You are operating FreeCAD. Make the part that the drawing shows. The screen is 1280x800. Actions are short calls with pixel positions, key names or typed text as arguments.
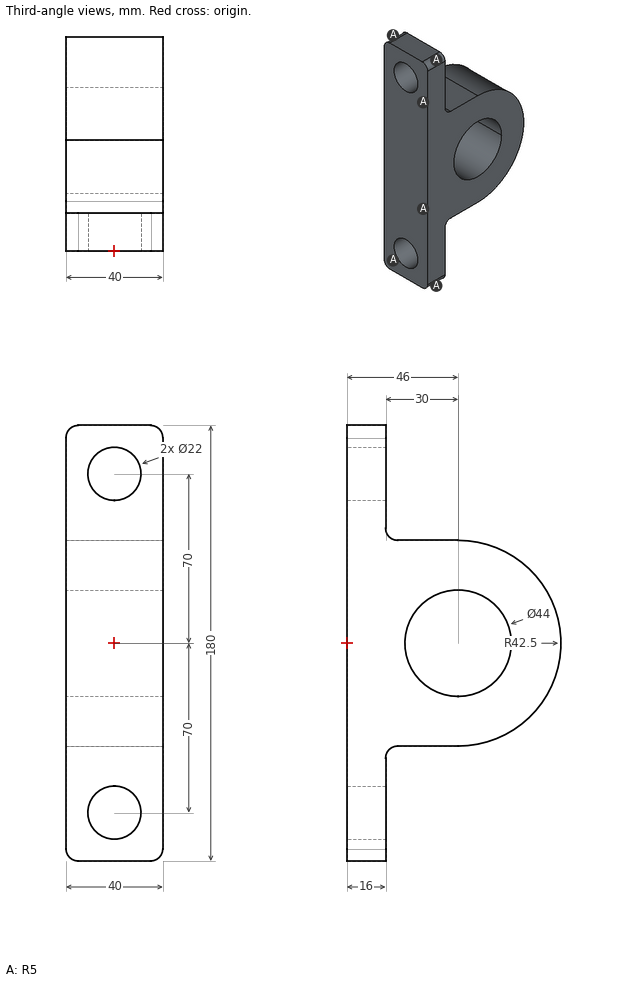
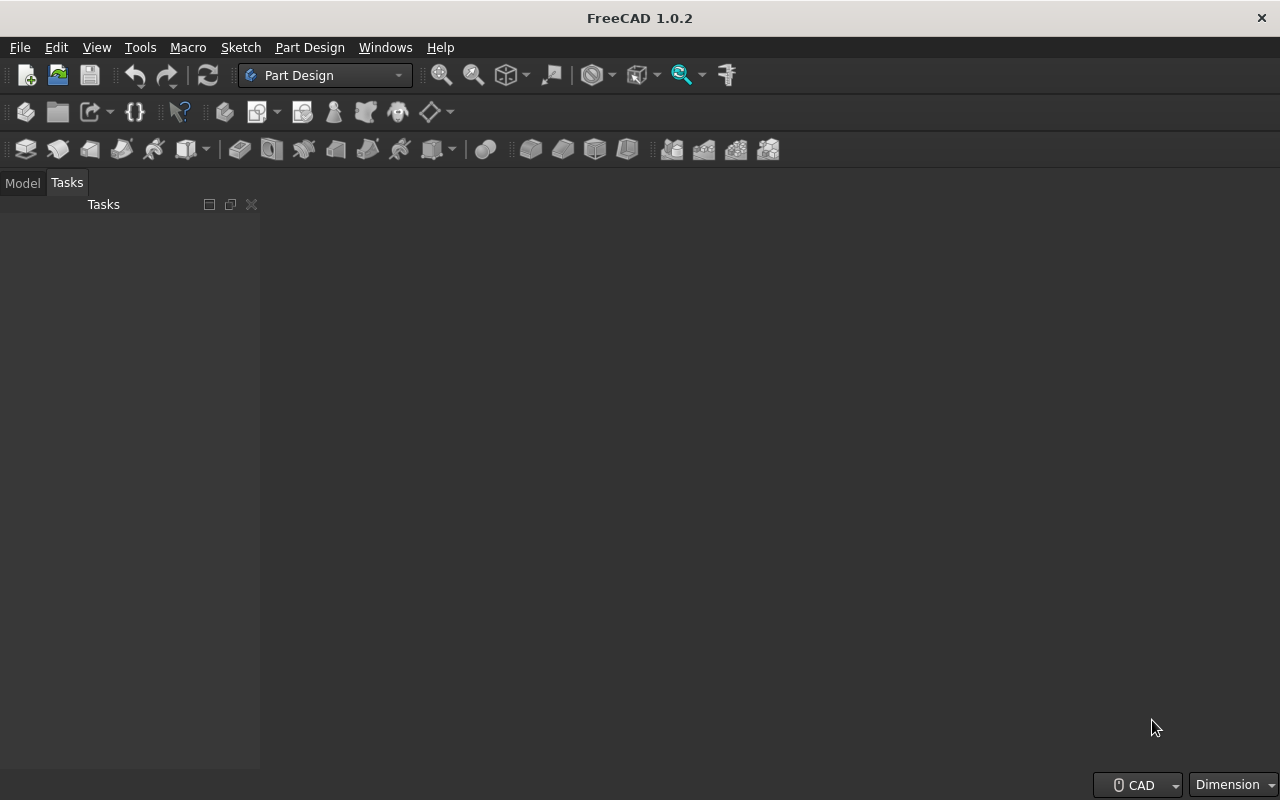
click(26, 76)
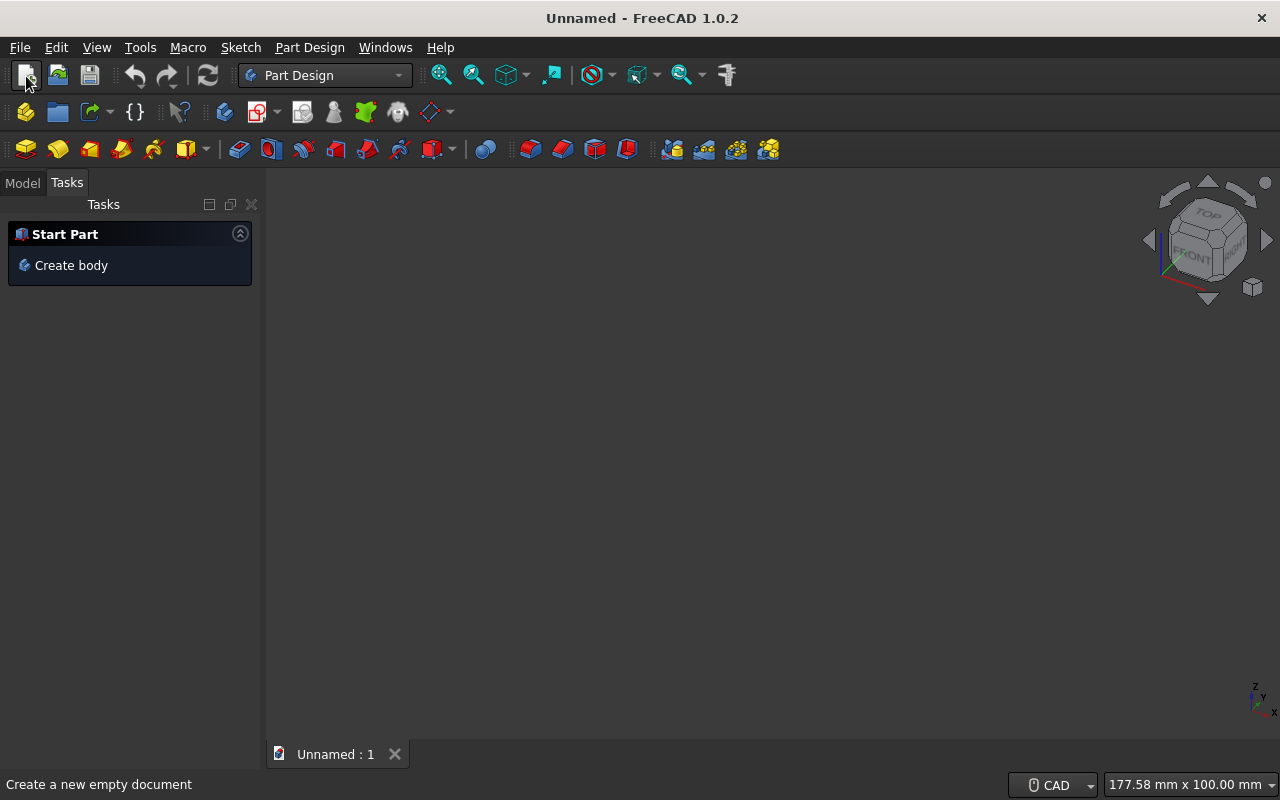
click(258, 112)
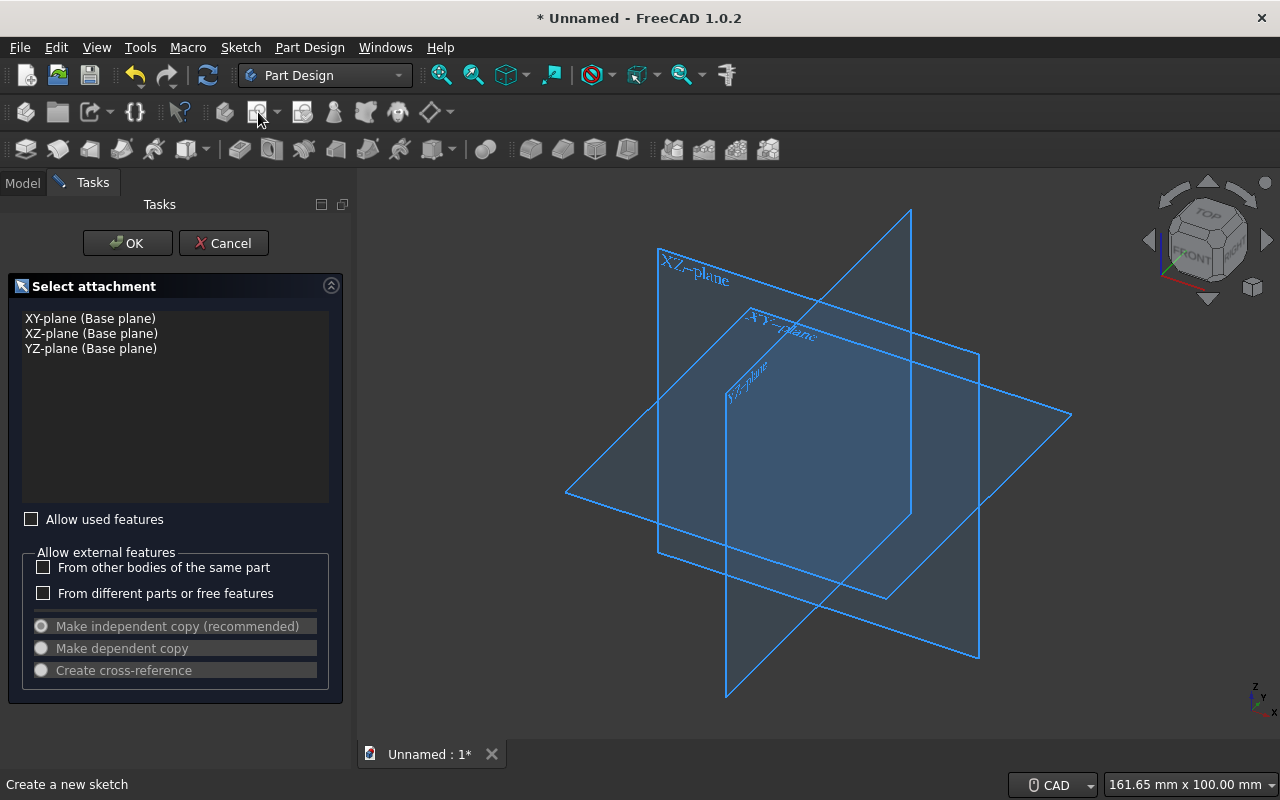
click(82, 334)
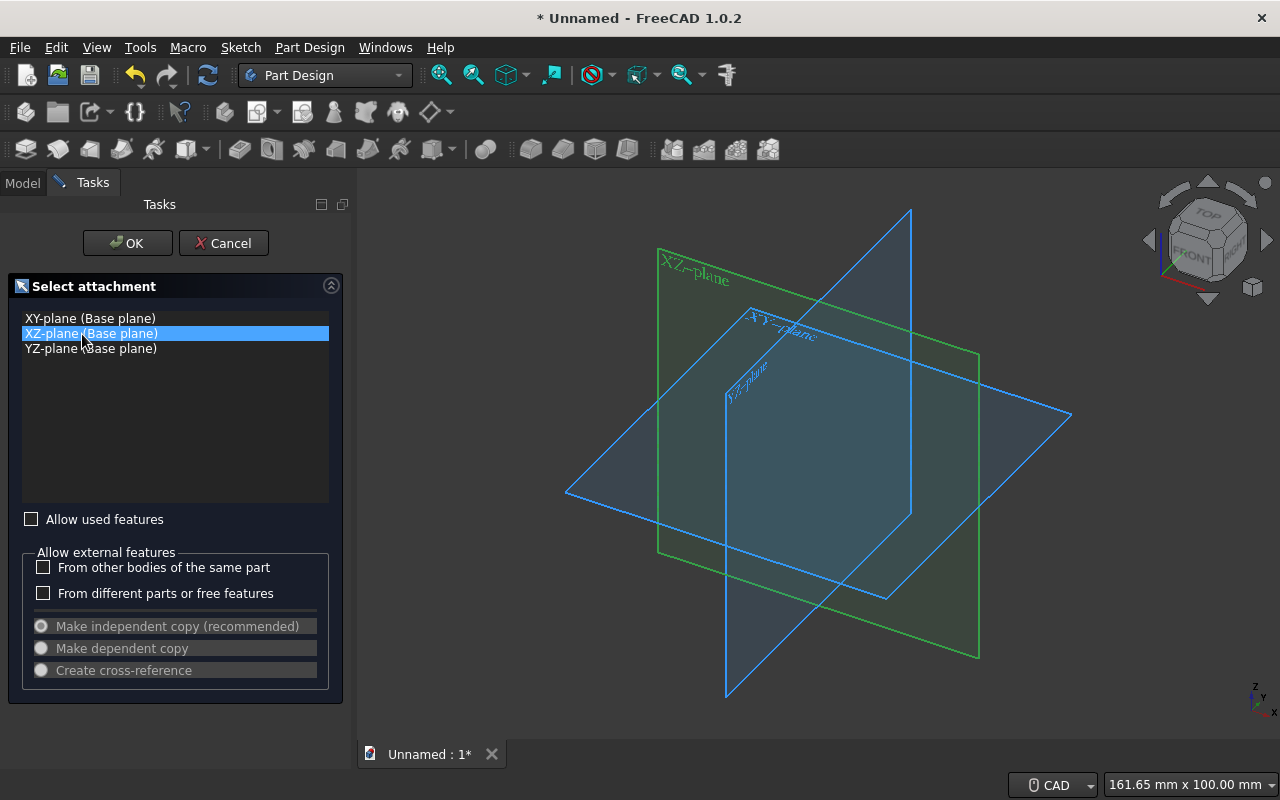
click(128, 243)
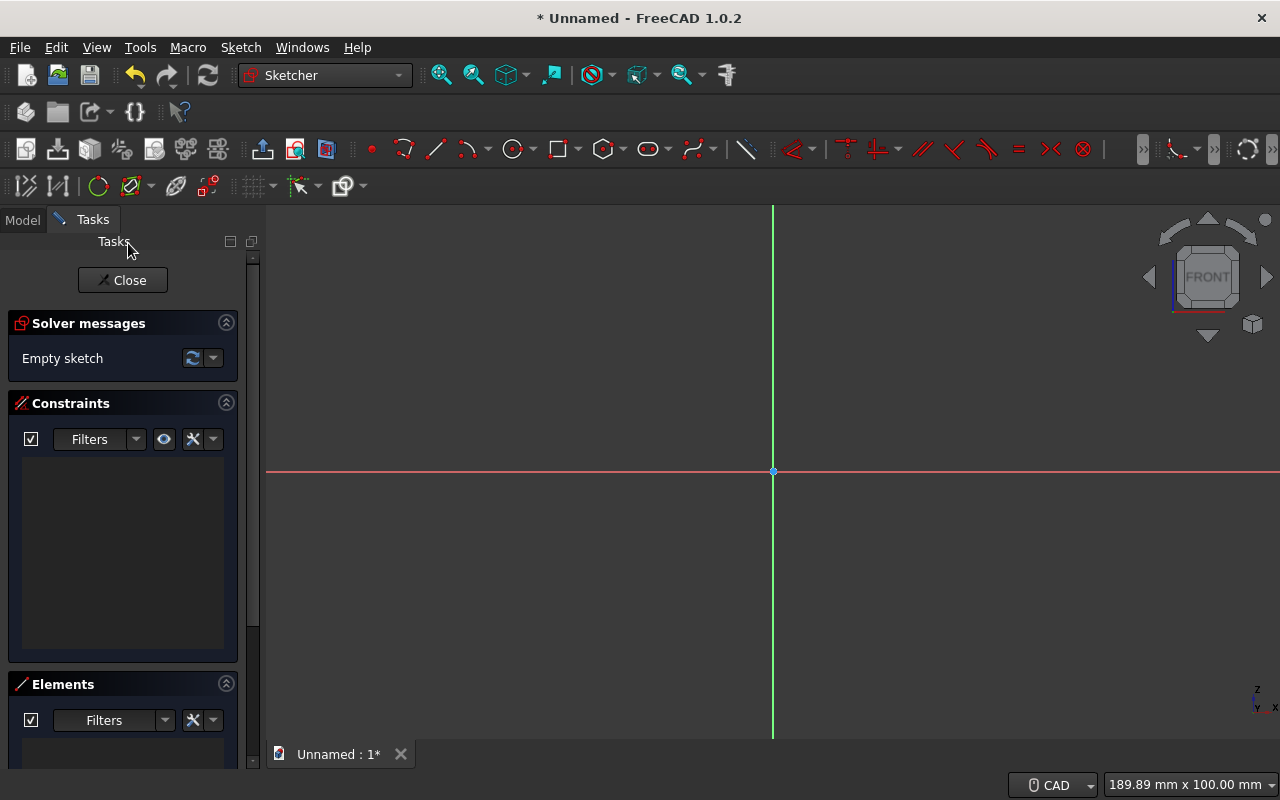
scroll(665, 472, down, 5)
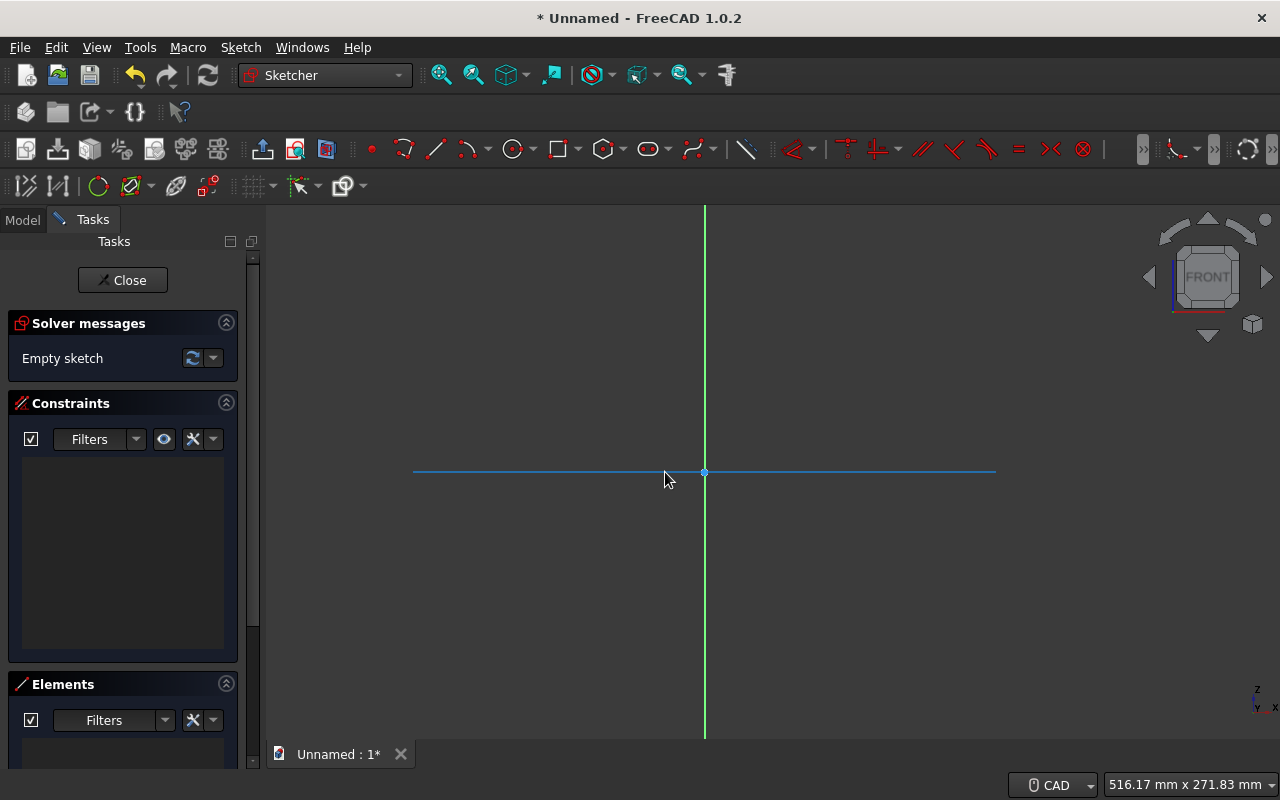
key(g)
key(v)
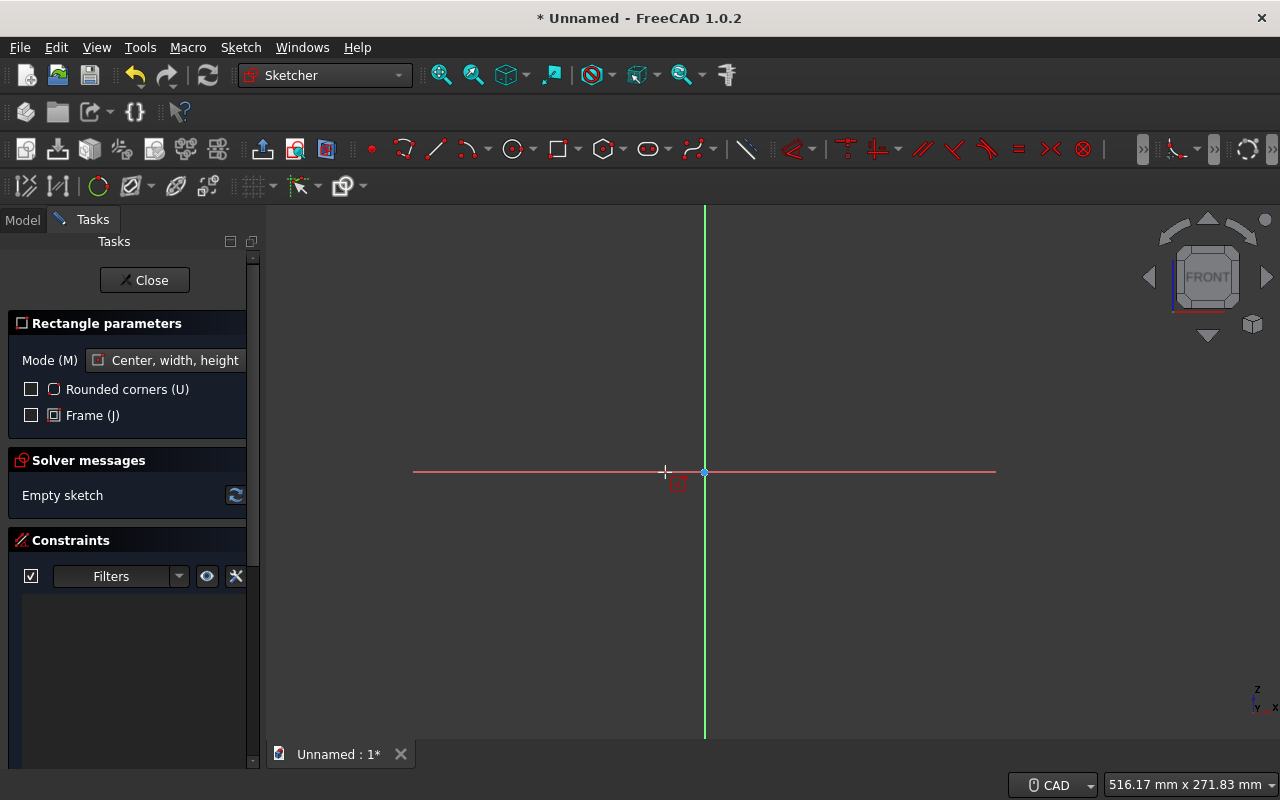
click(705, 472)
click(744, 296)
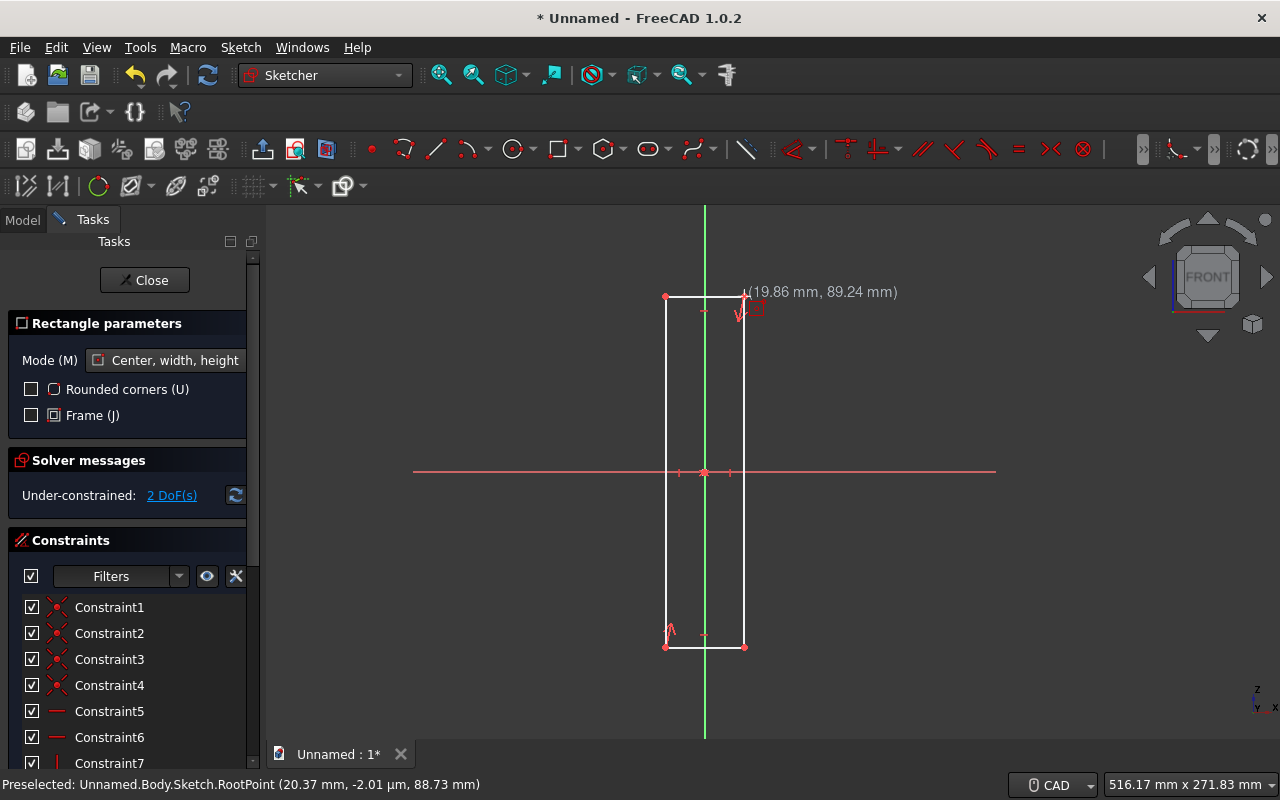
key(g)
key(c)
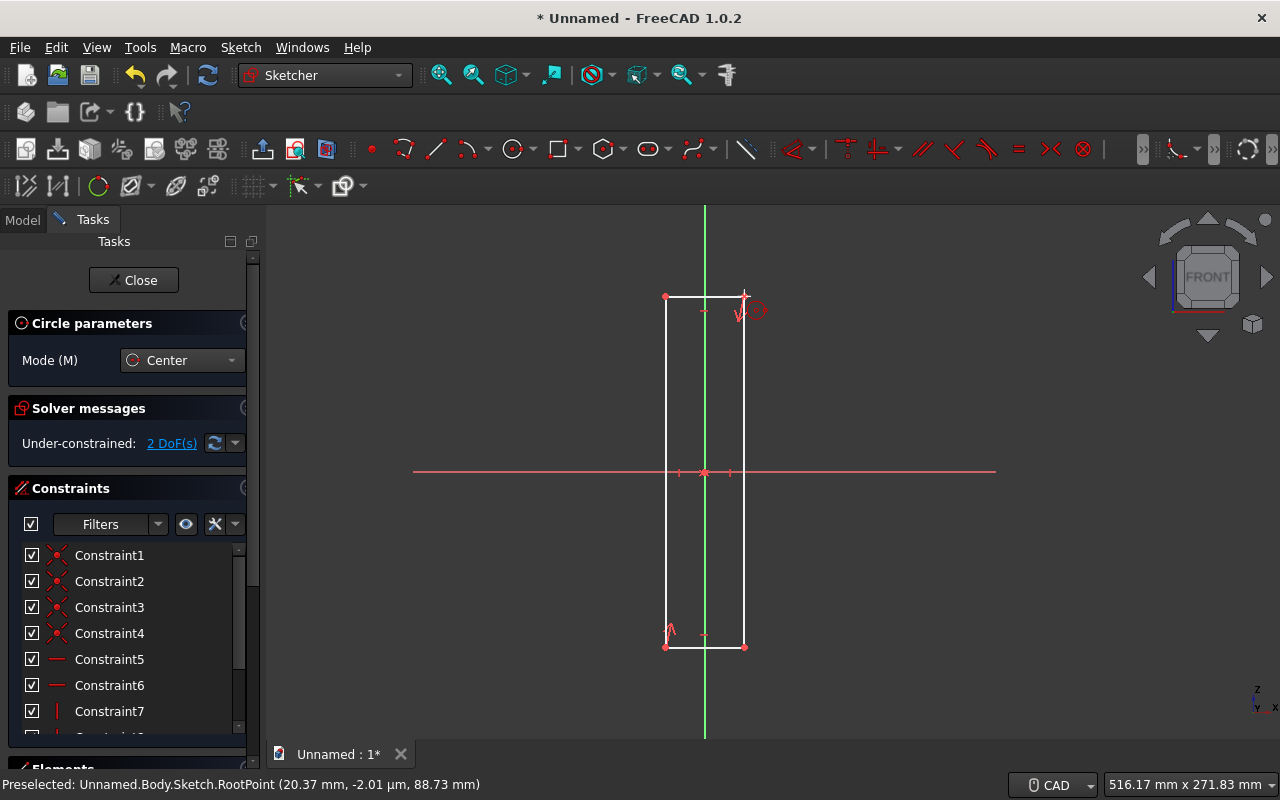
click(705, 335)
click(720, 320)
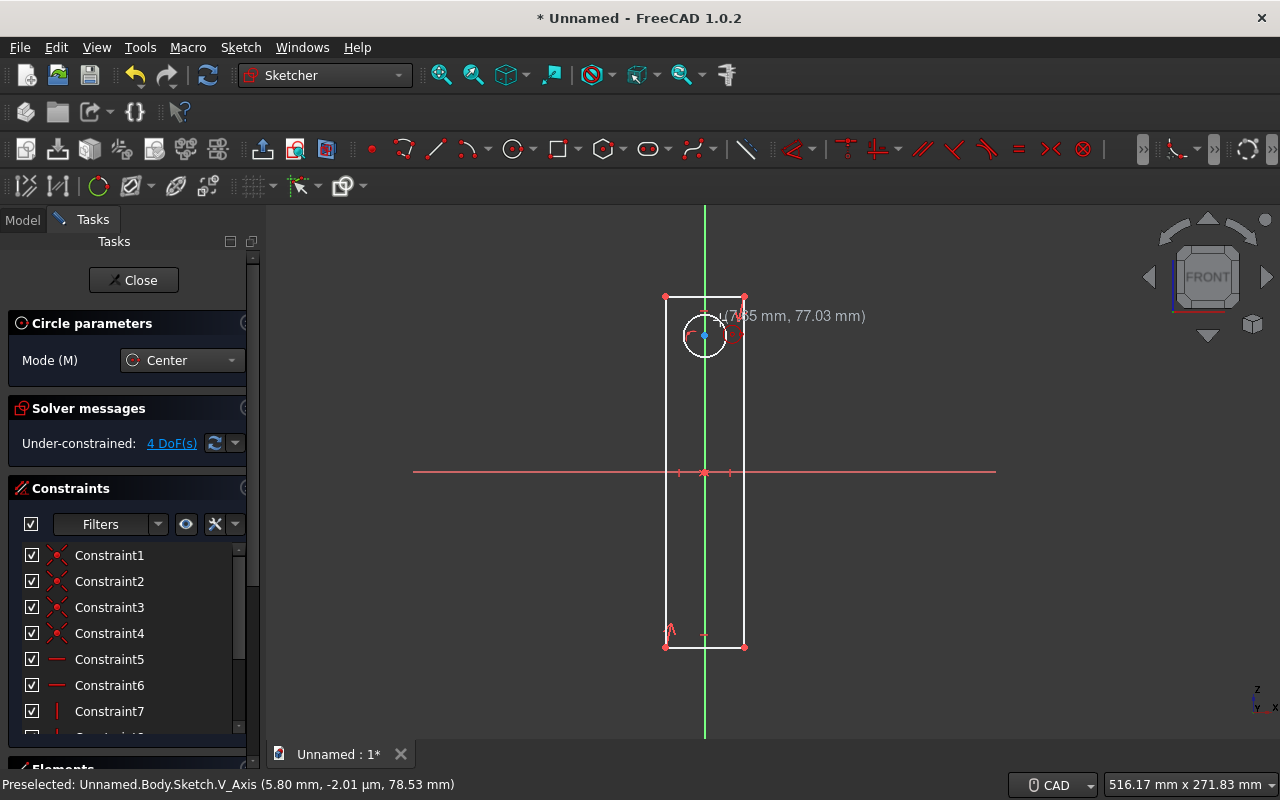
click(705, 610)
click(720, 595)
key(Escape)